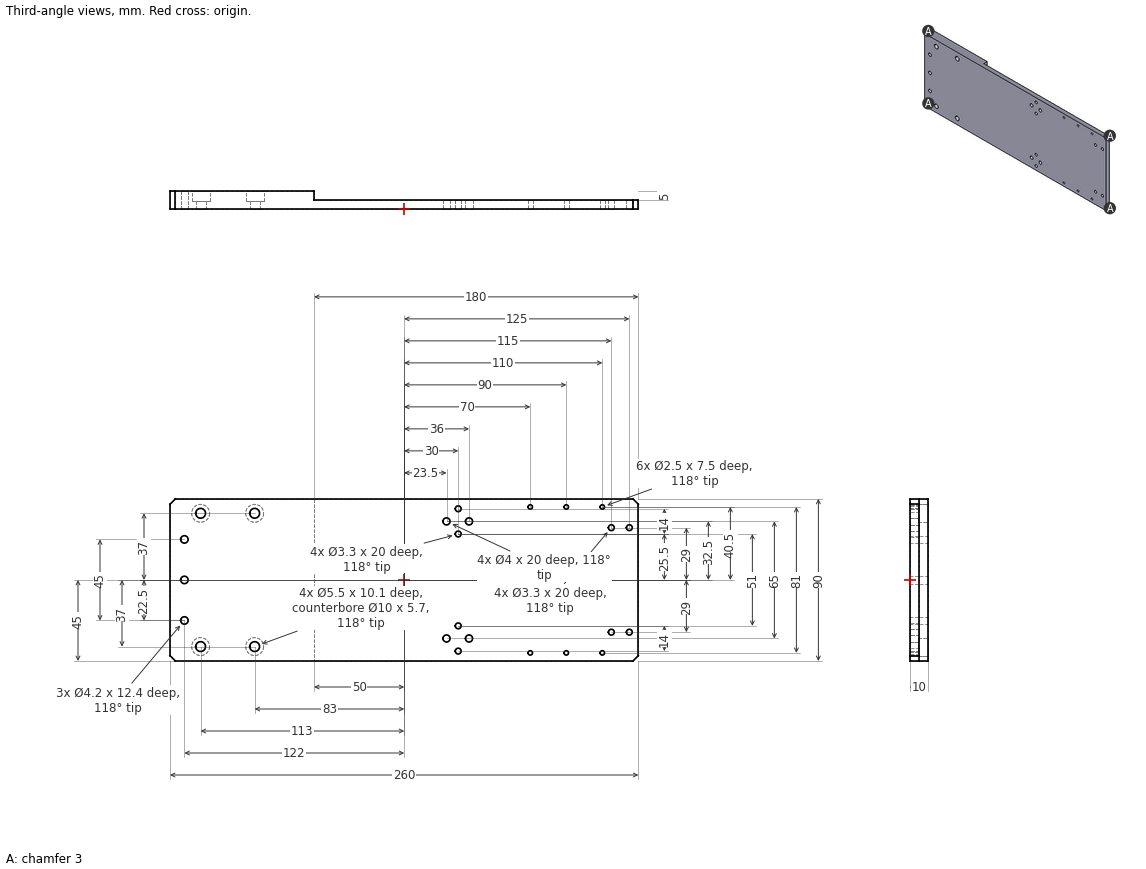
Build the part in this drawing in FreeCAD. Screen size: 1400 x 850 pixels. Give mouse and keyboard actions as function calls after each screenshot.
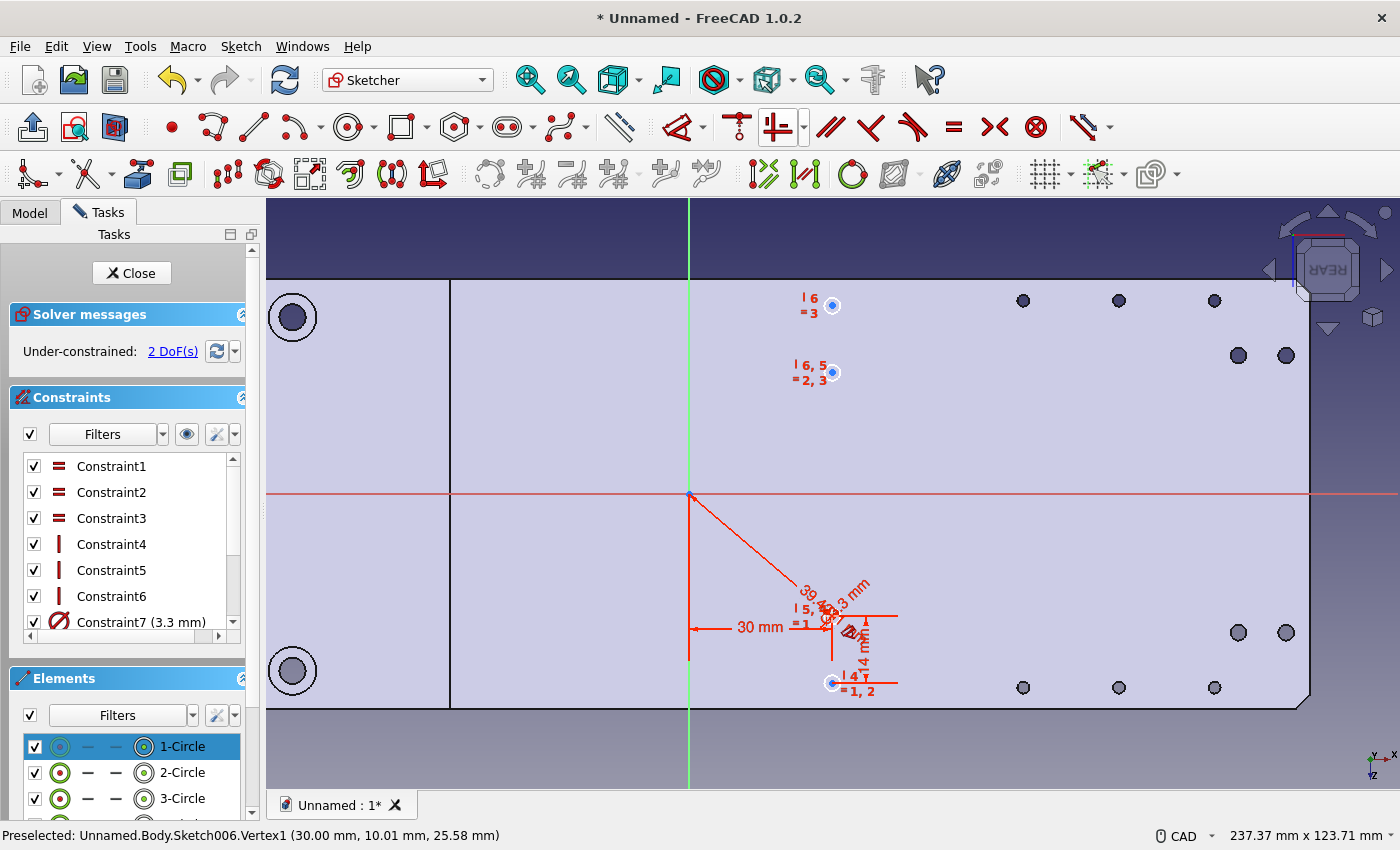
click(832, 373)
click(866, 439)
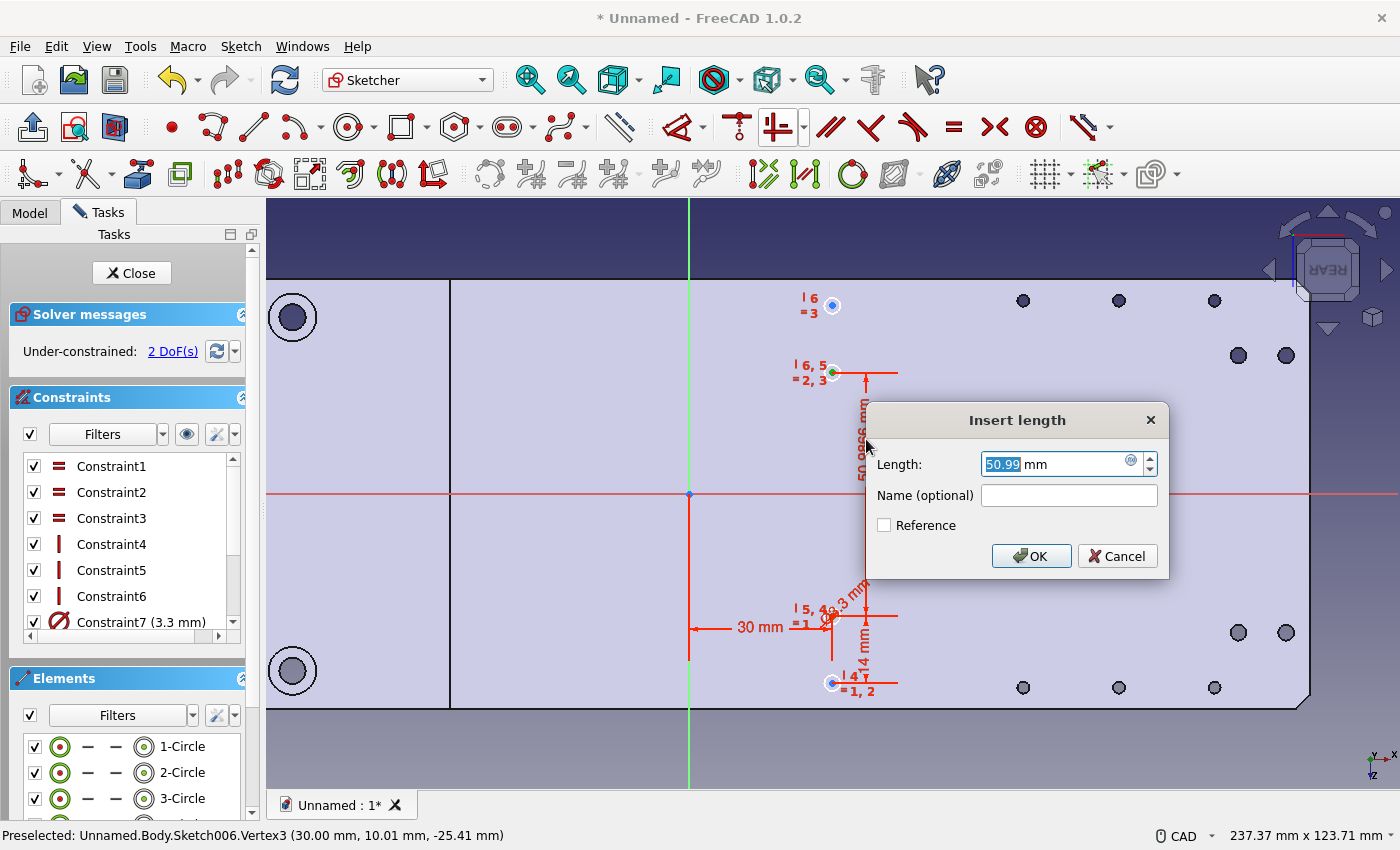
text(51)
key(Return)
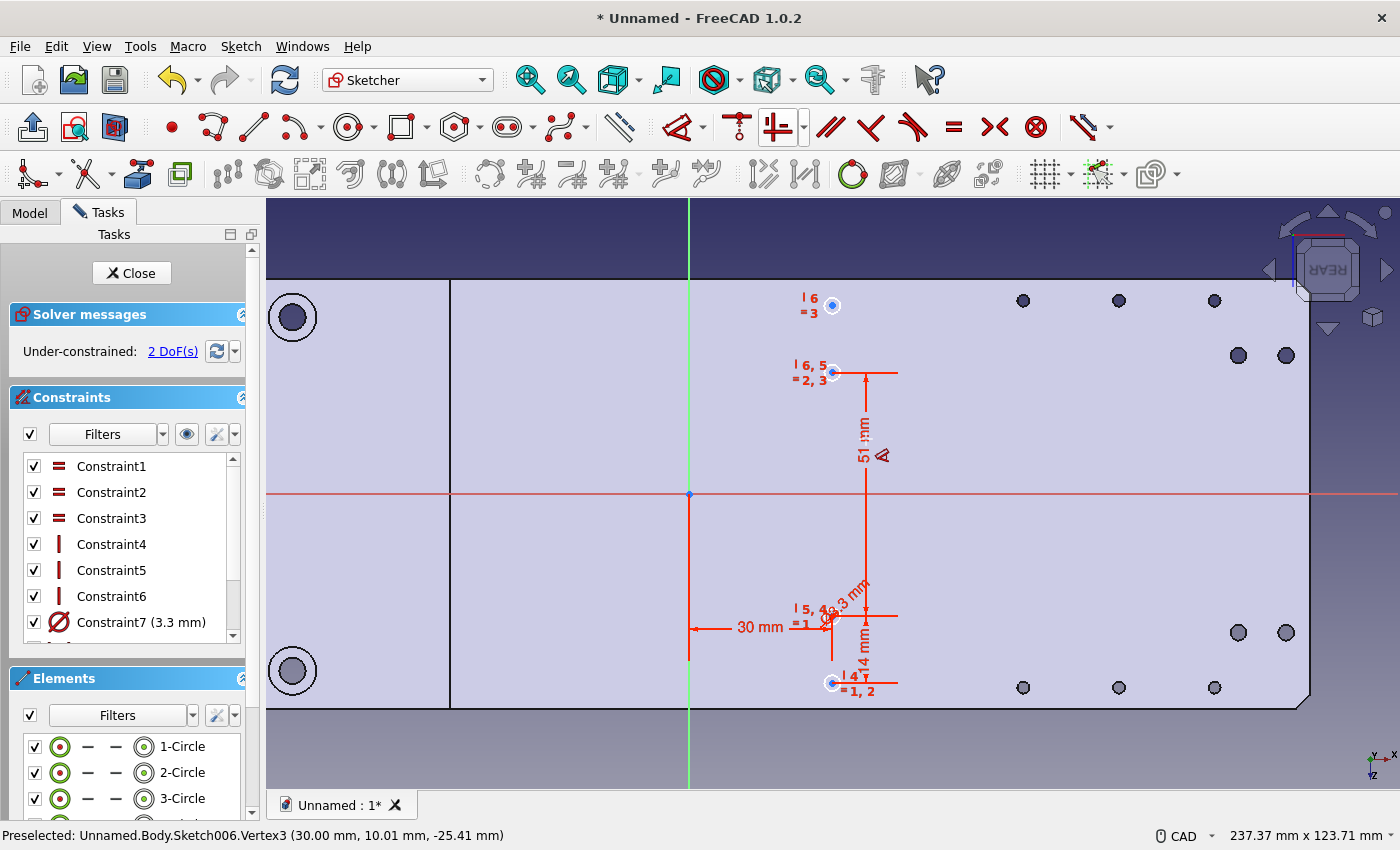
click(832, 373)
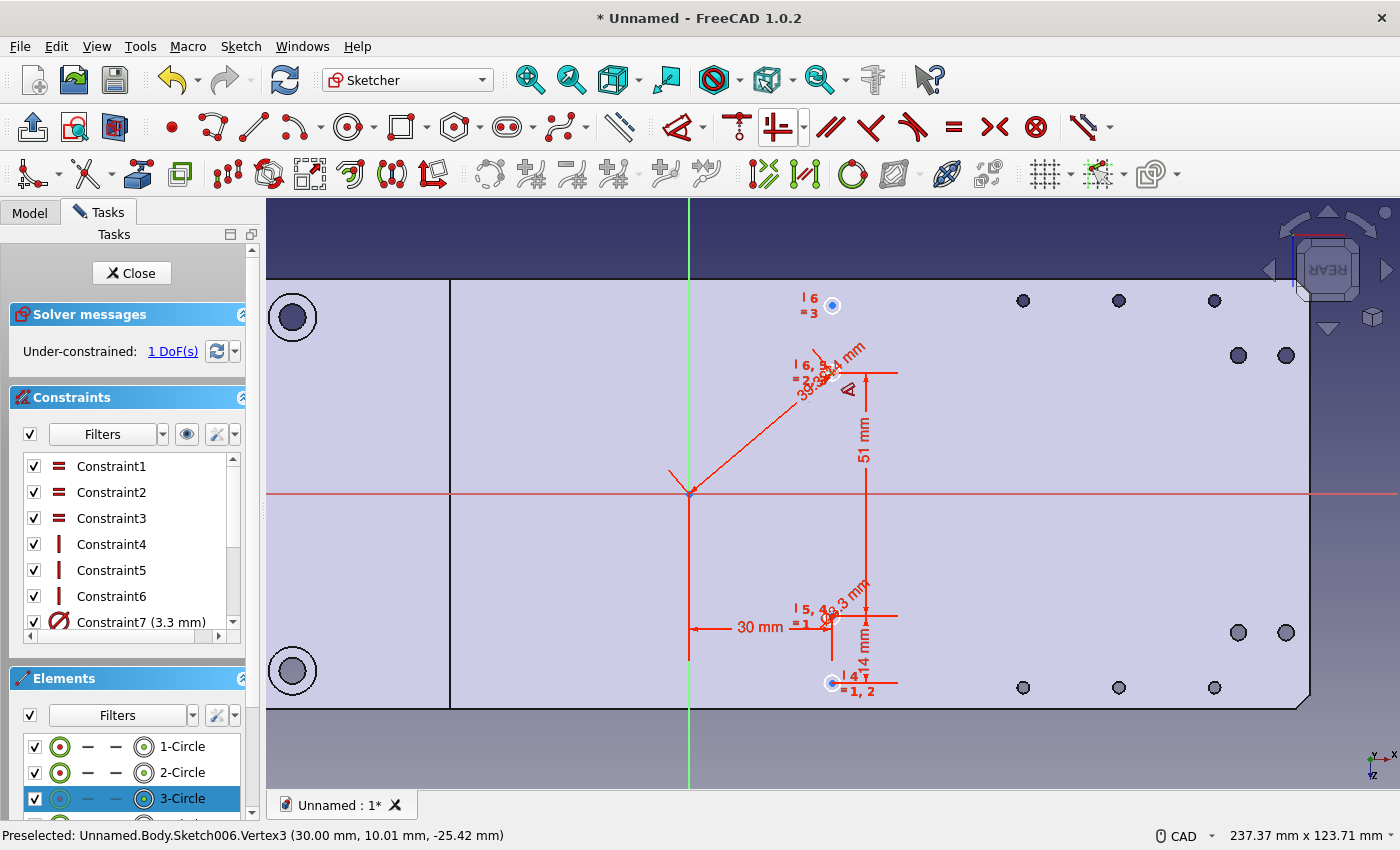
click(832, 306)
click(866, 339)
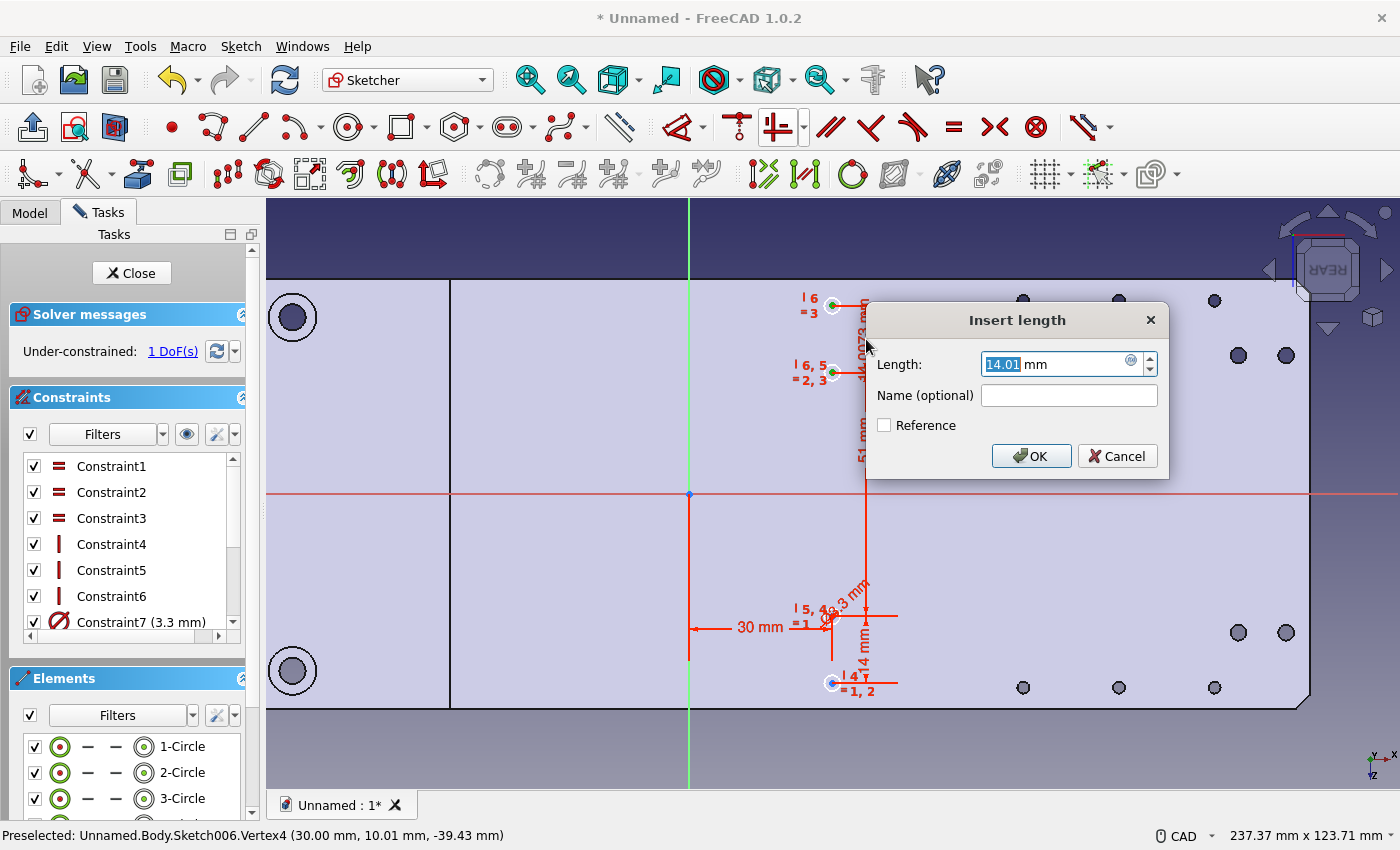
text(14)
key(Return)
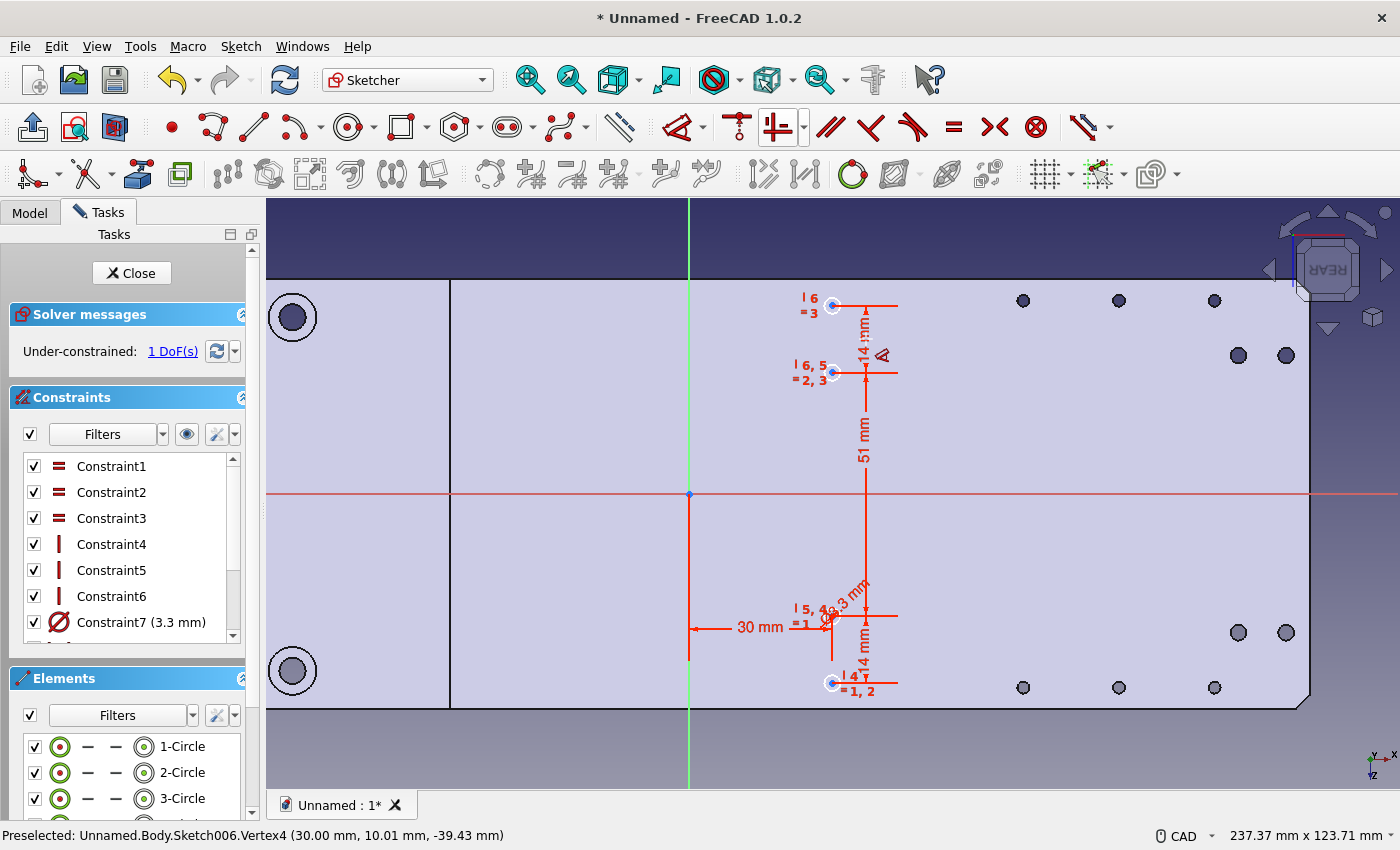
click(832, 616)
click(655, 555)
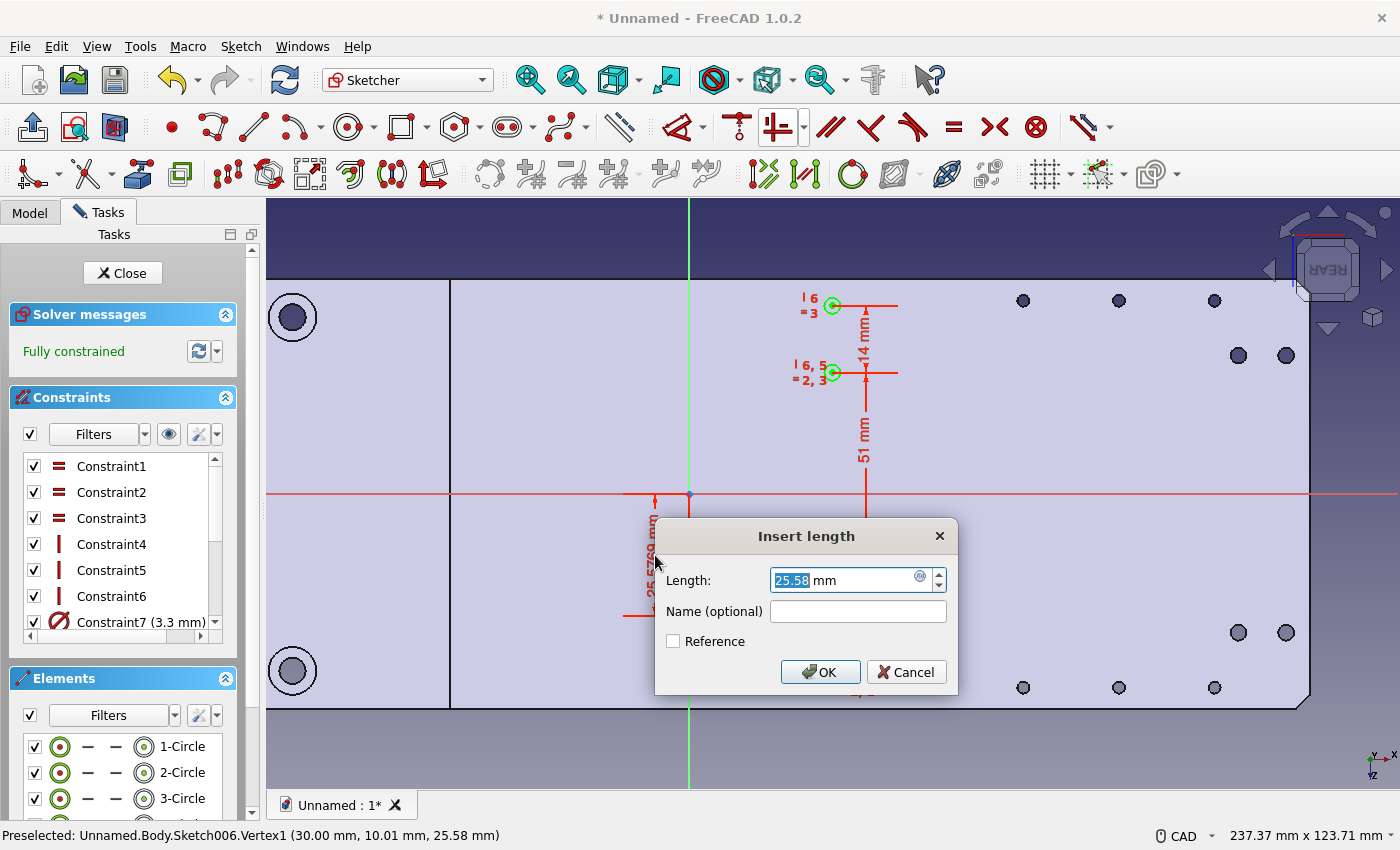
text(25.5)
key(Return)
key(Escape)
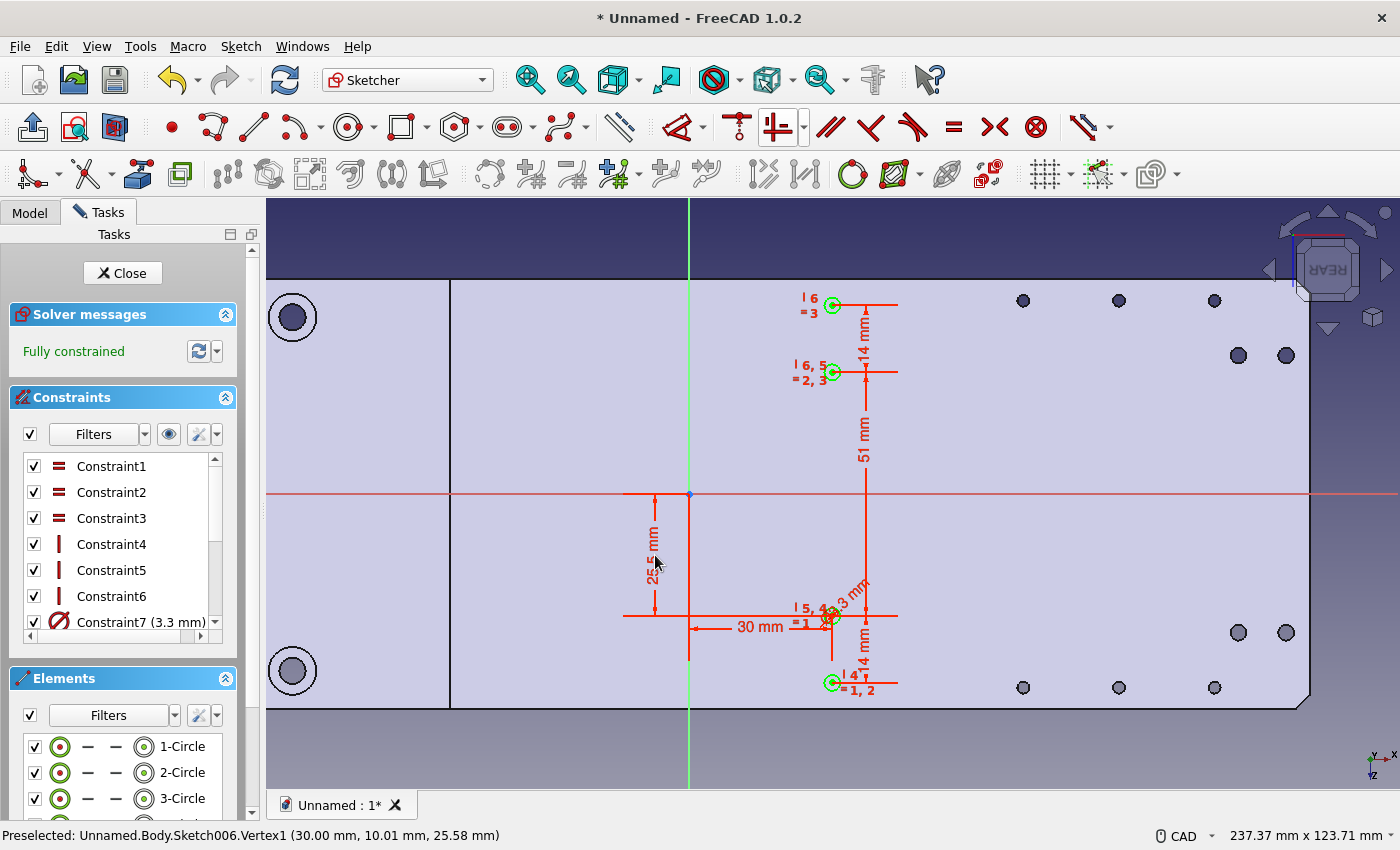
click(123, 273)